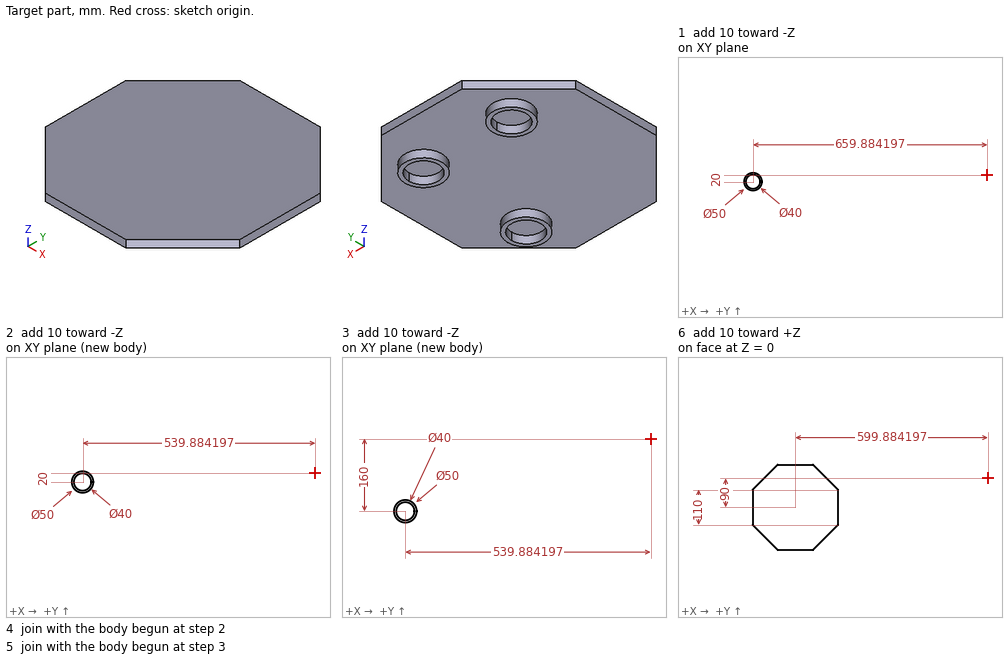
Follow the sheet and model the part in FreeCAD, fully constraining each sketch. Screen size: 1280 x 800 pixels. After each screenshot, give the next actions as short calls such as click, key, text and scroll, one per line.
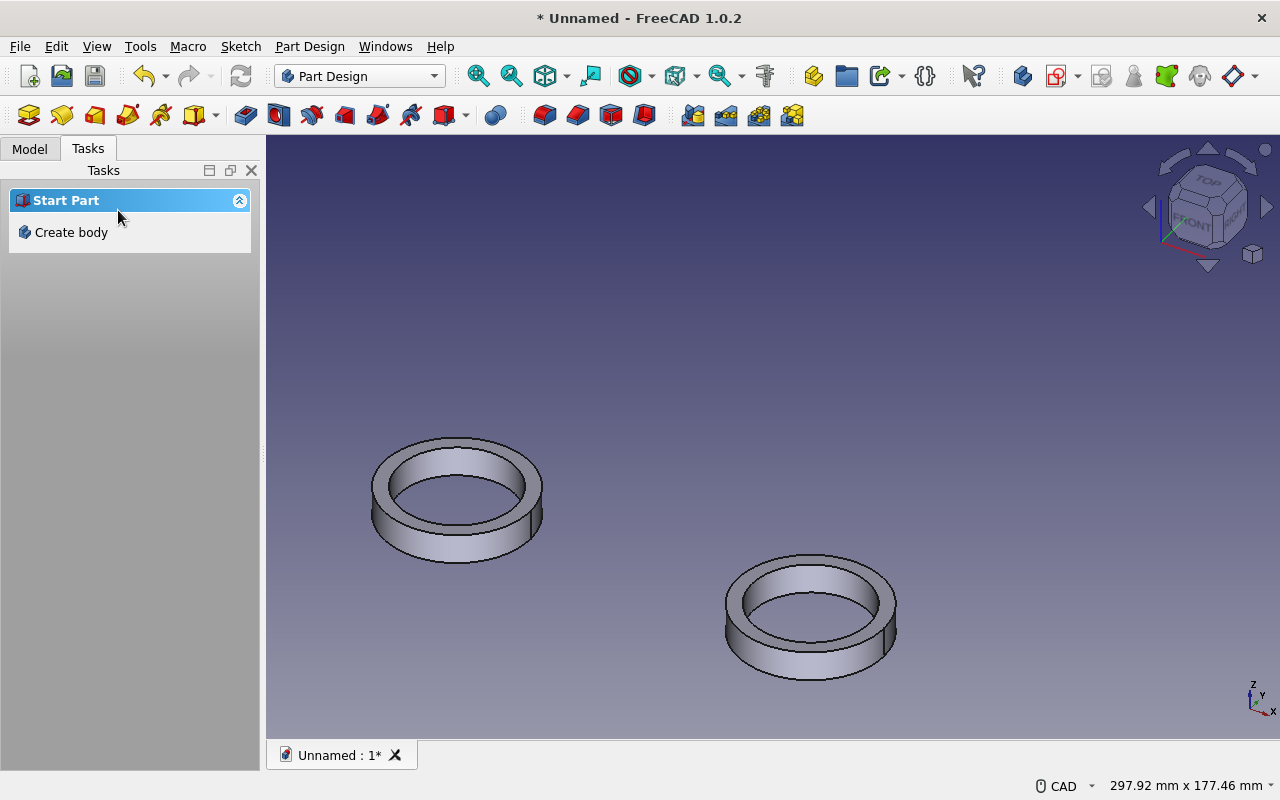
key(v)
key(f)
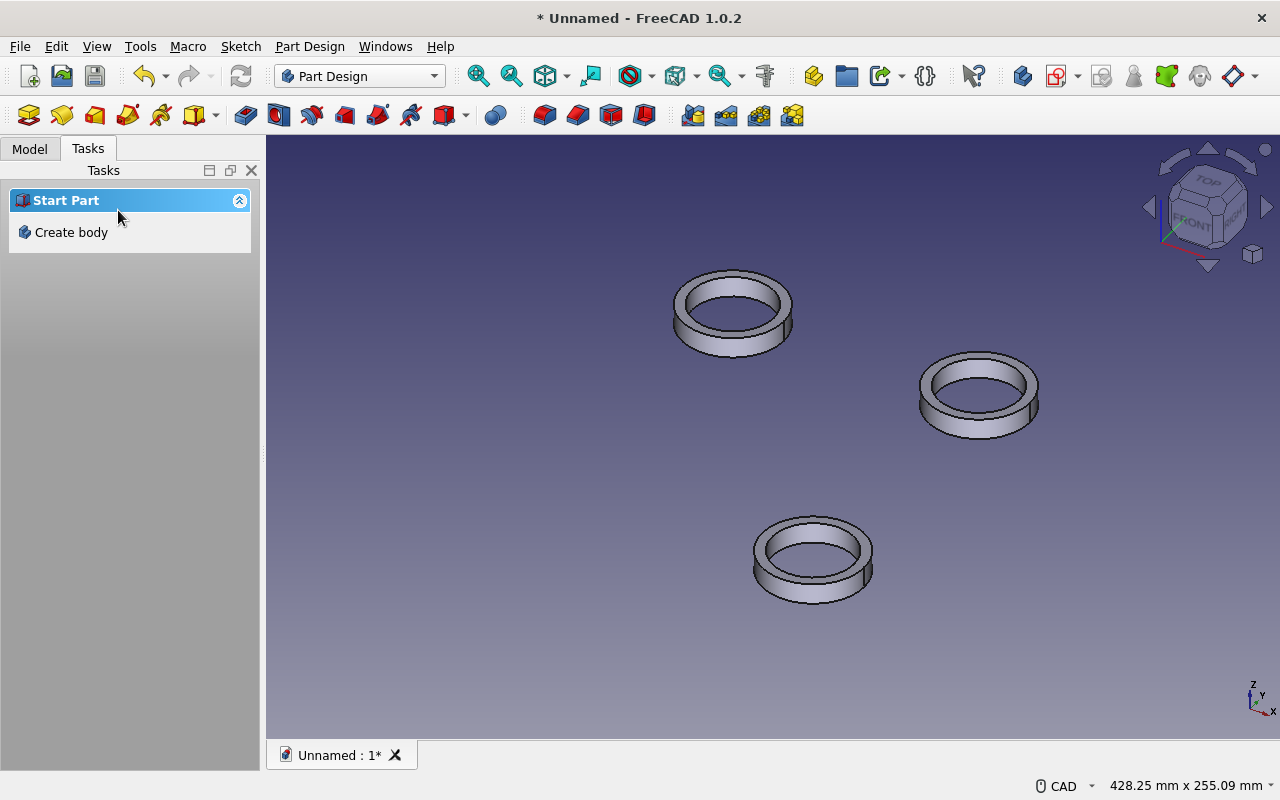
click(30, 148)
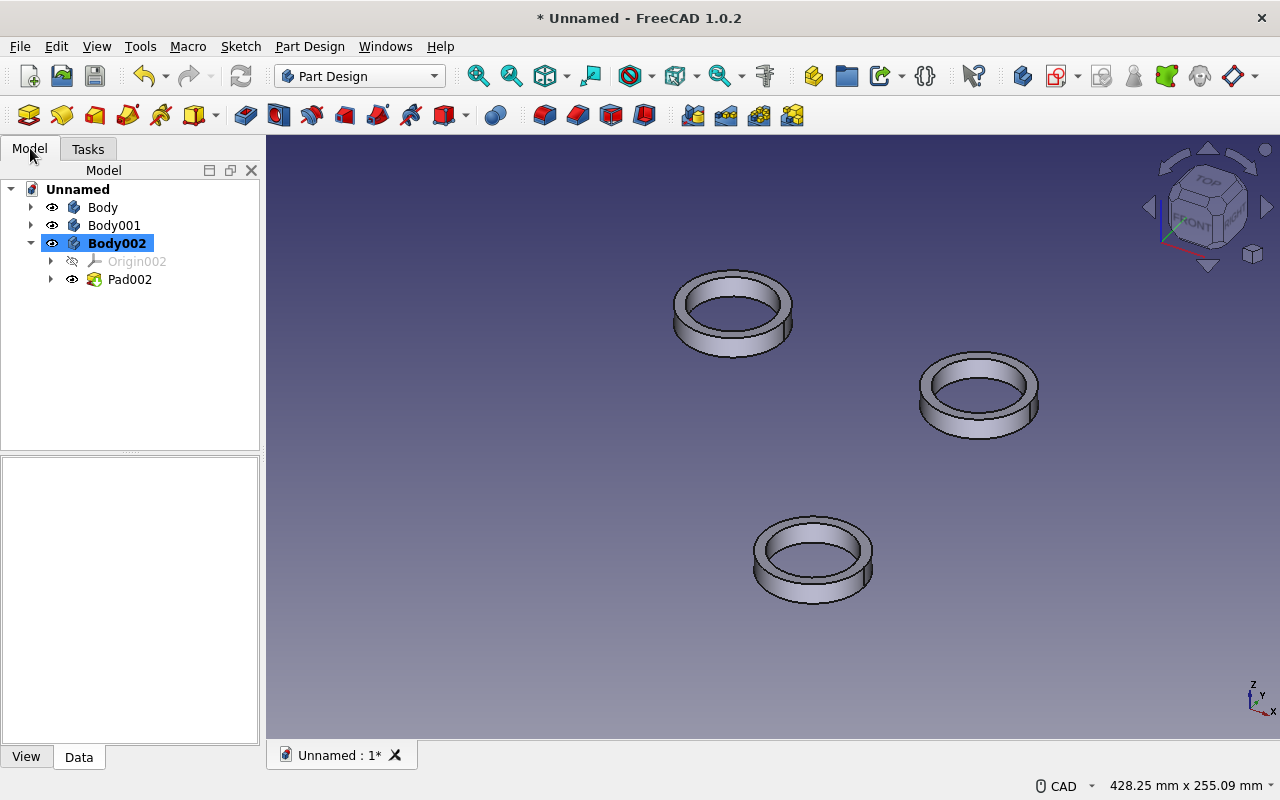
double_click(97, 207)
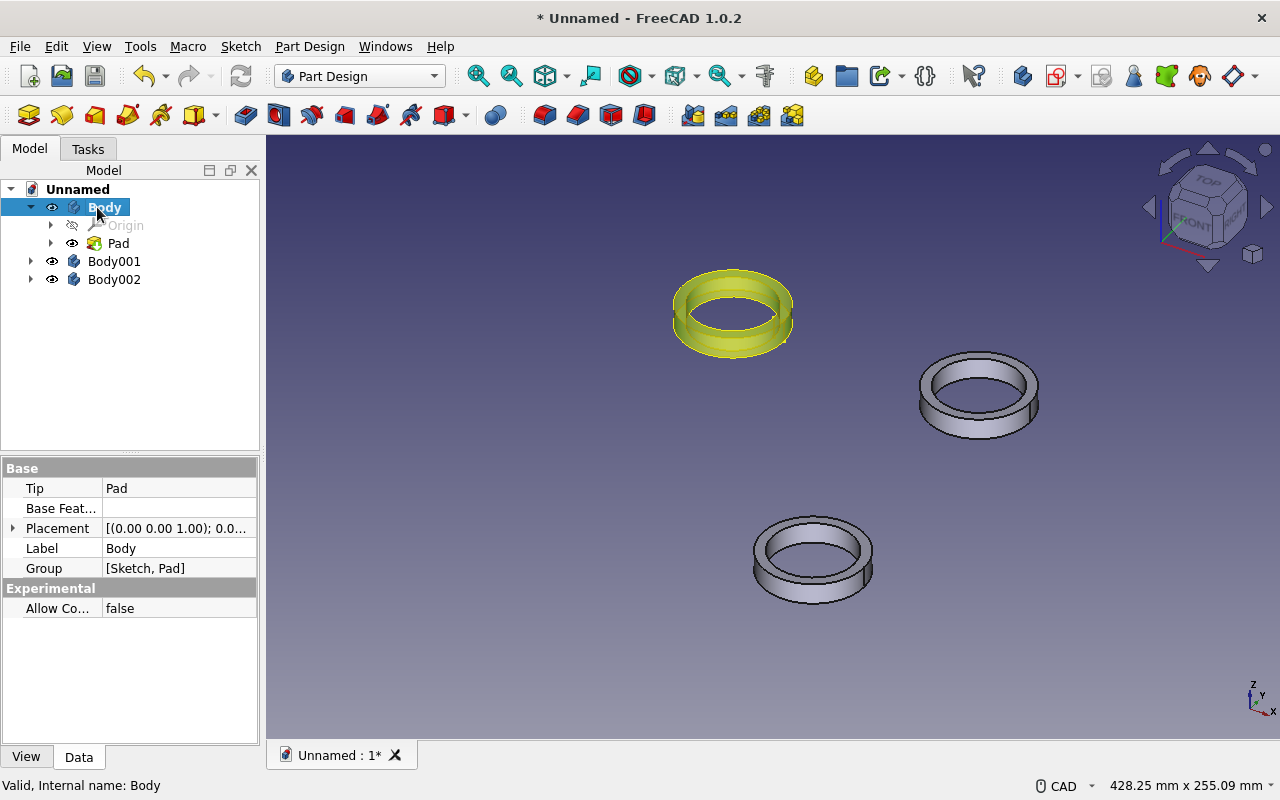
click(97, 207)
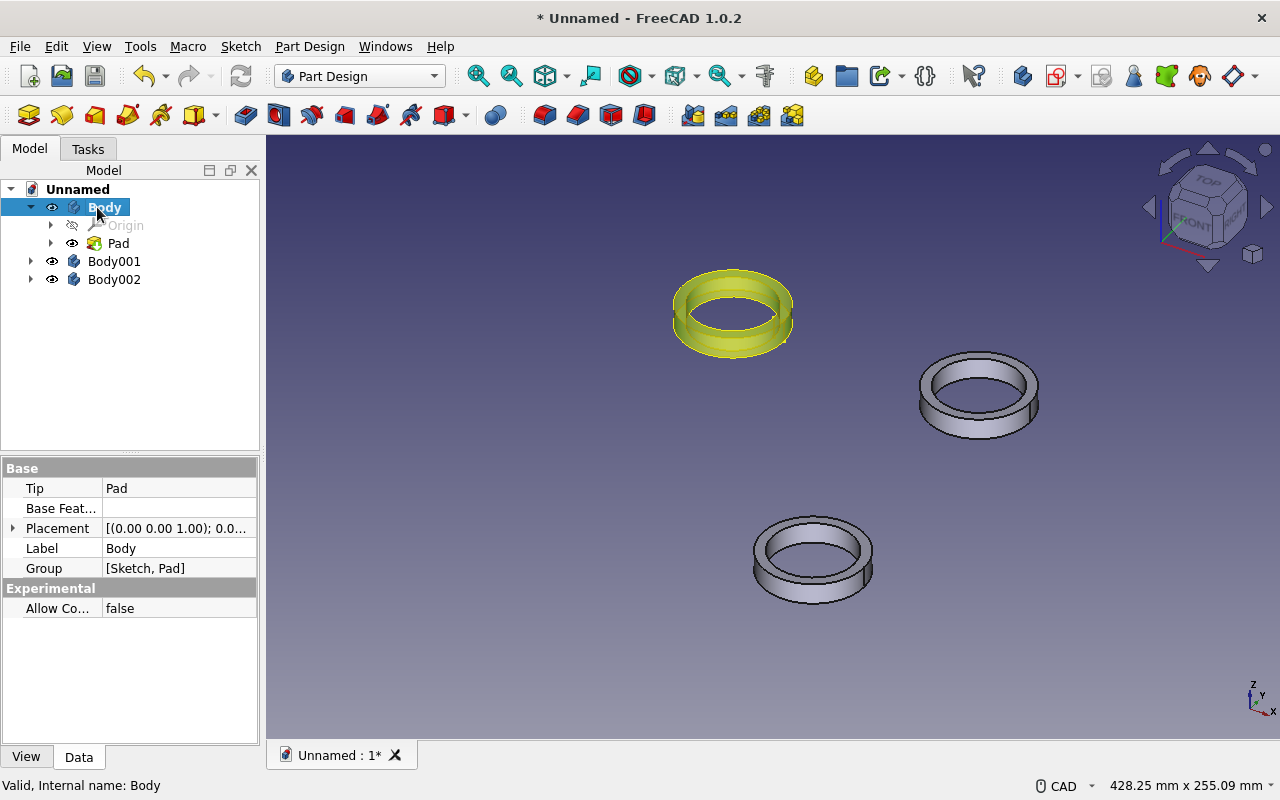
click(148, 608)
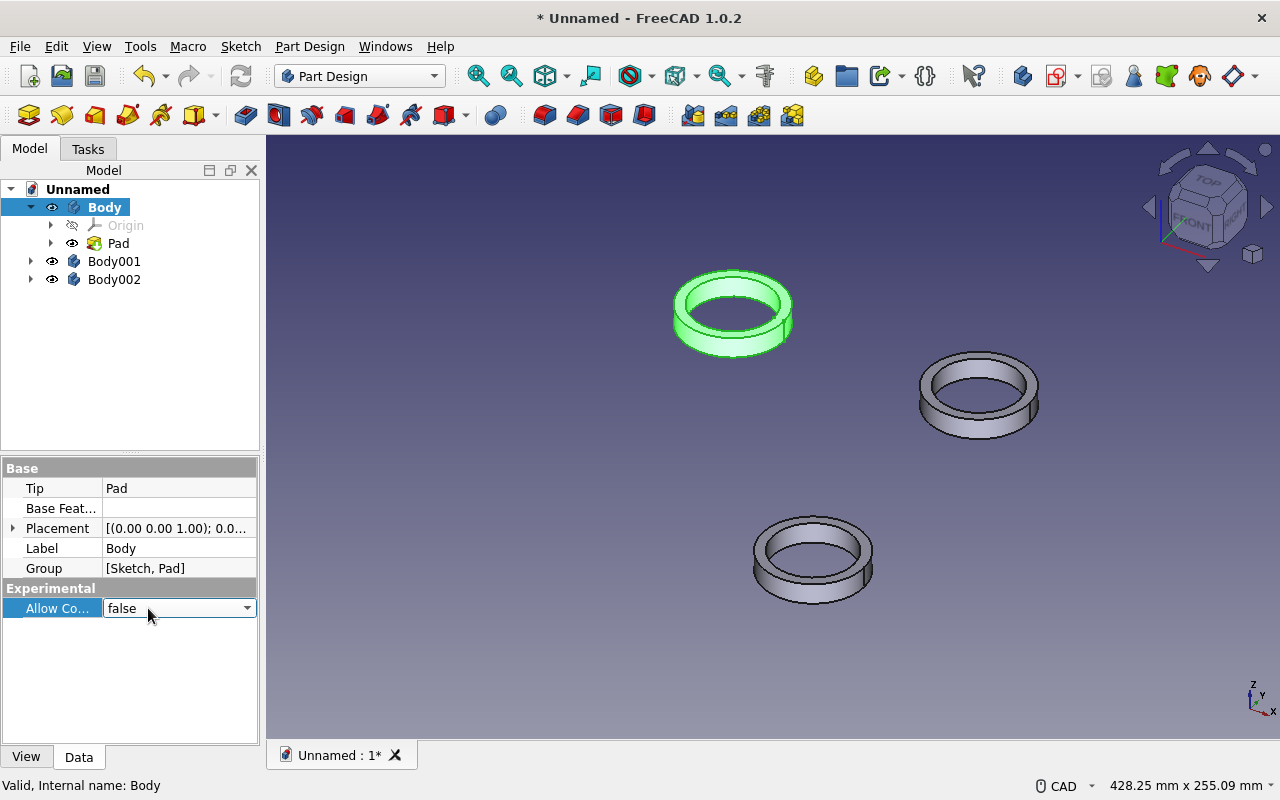
click(148, 608)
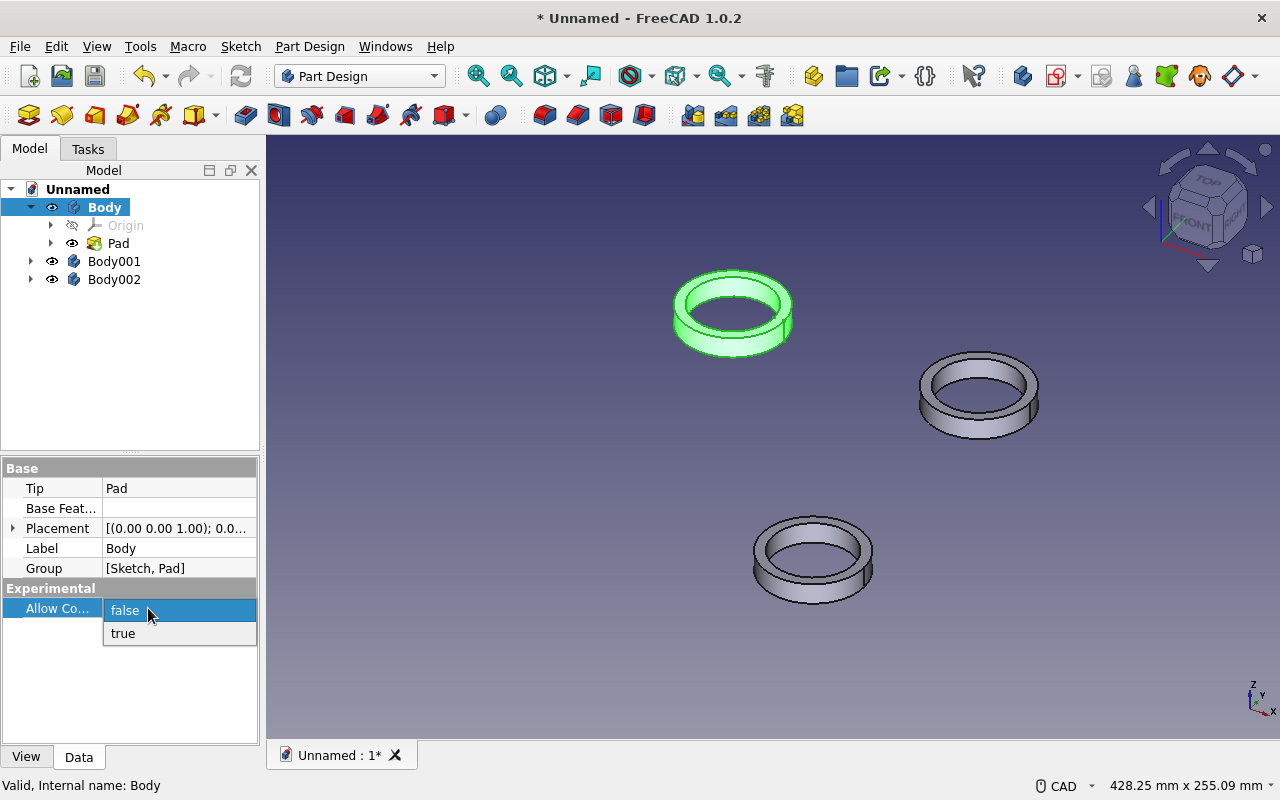
click(178, 634)
key(Return)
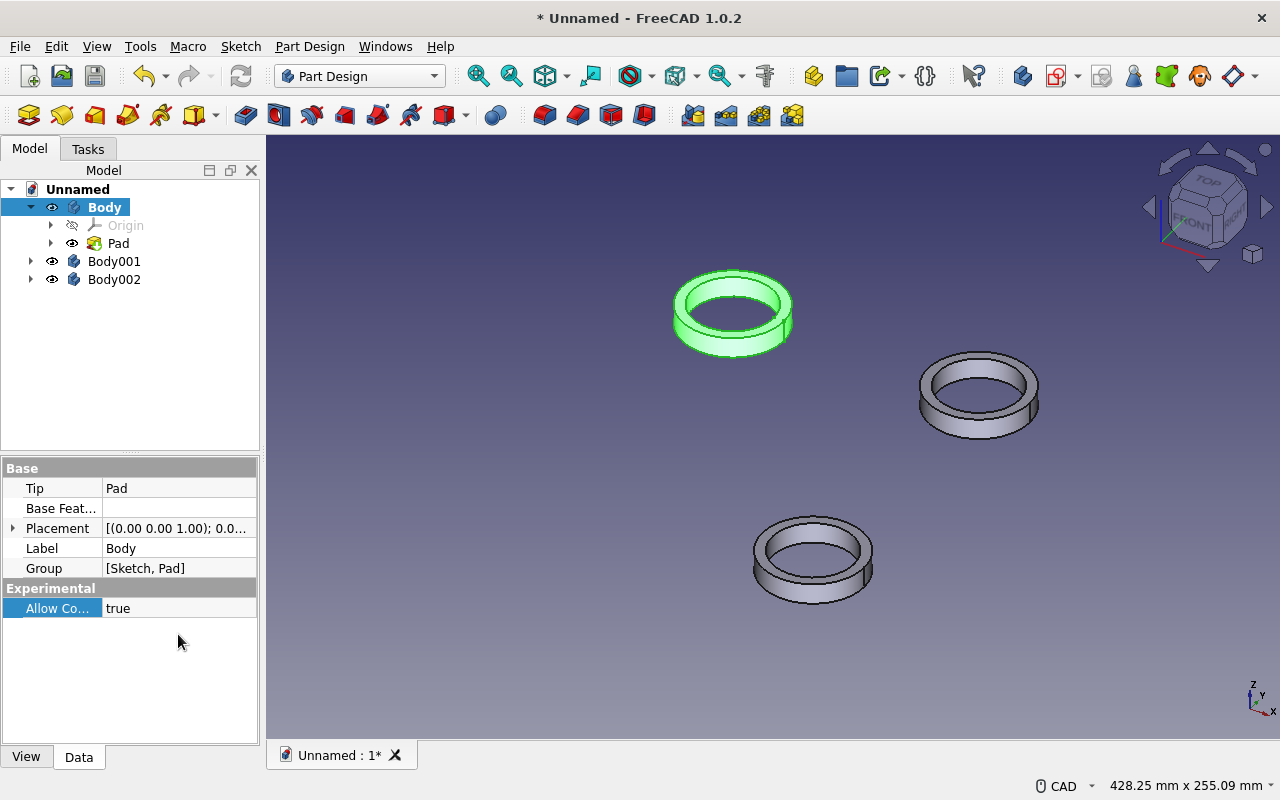
click(97, 261)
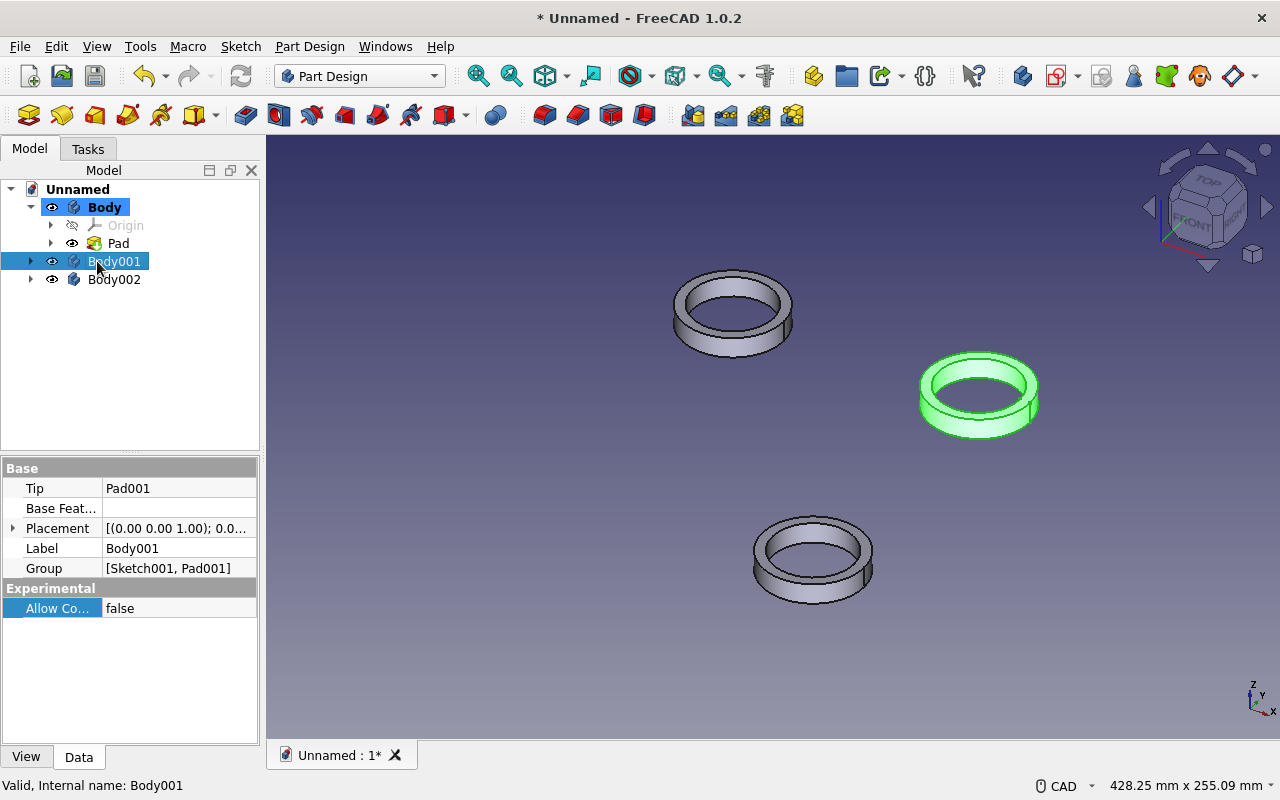
click(496, 116)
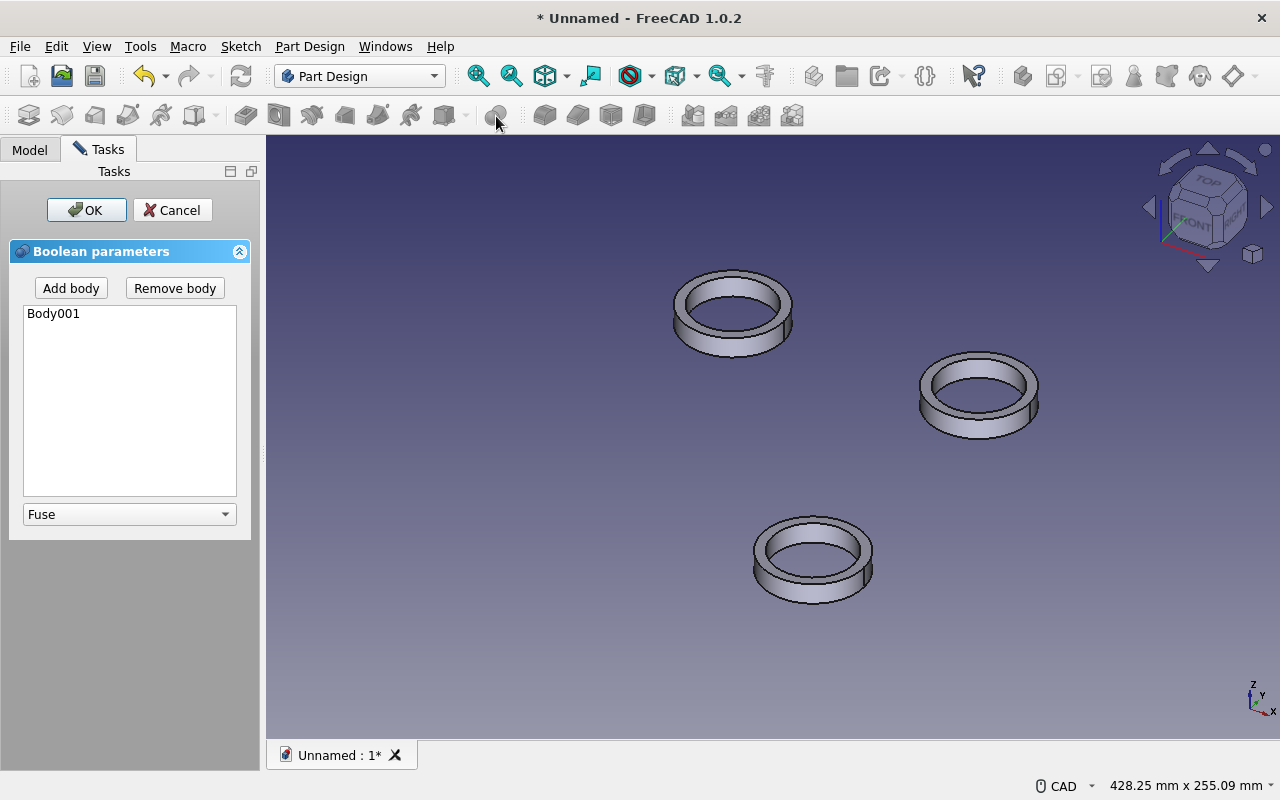
click(87, 210)